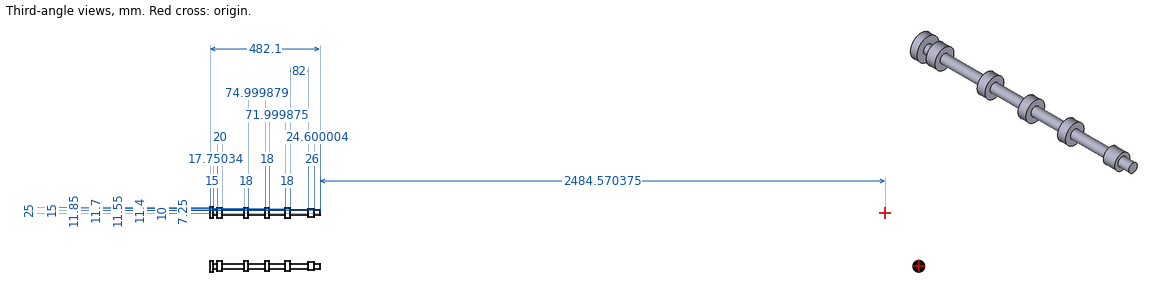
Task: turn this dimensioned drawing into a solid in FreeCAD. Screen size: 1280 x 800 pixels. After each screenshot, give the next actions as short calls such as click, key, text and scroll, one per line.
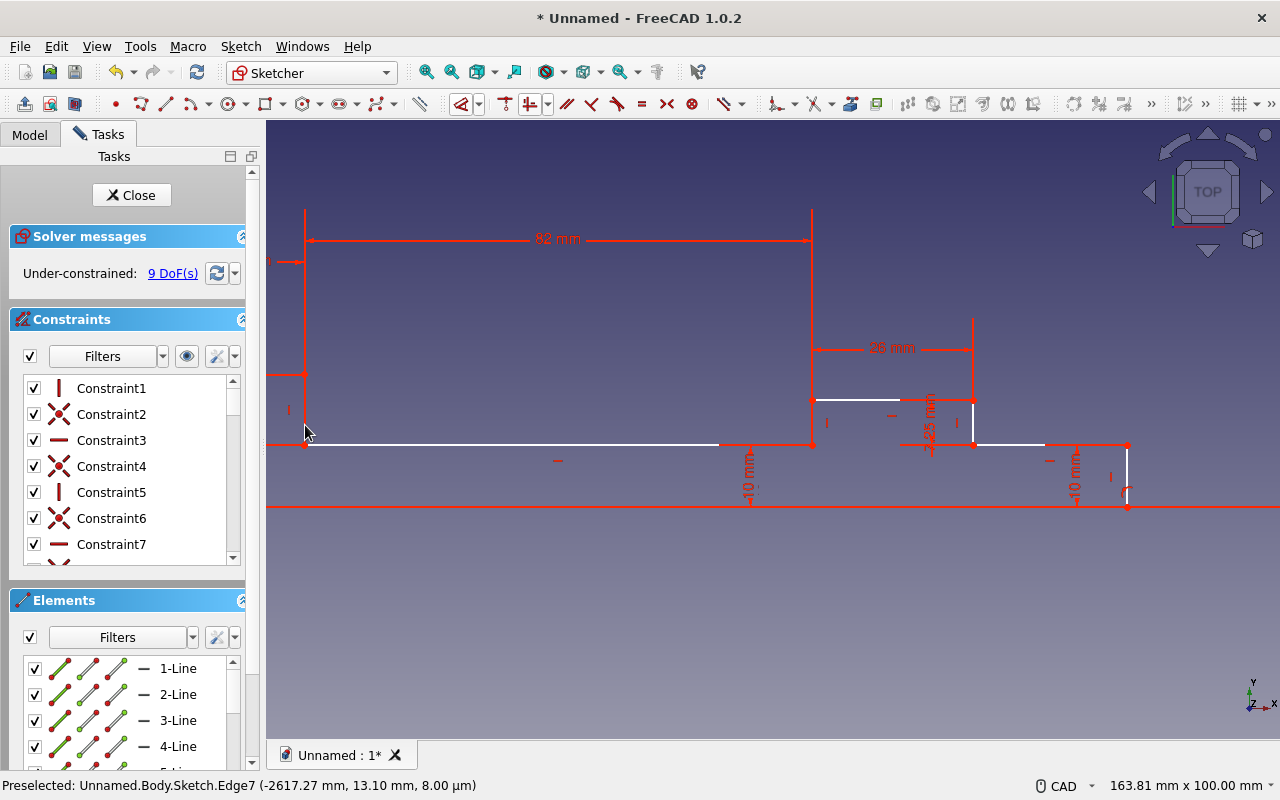
scroll(975, 429, down, 8)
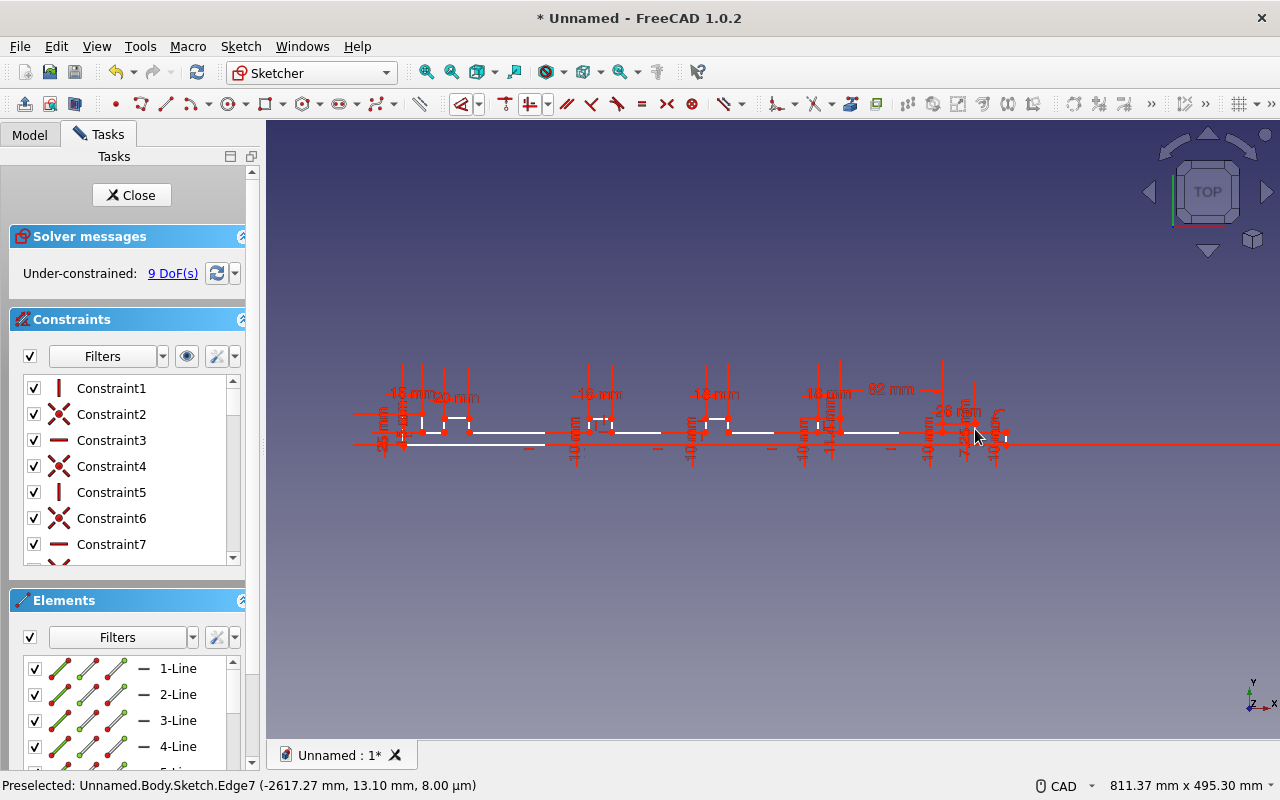
scroll(612, 429, up, 7)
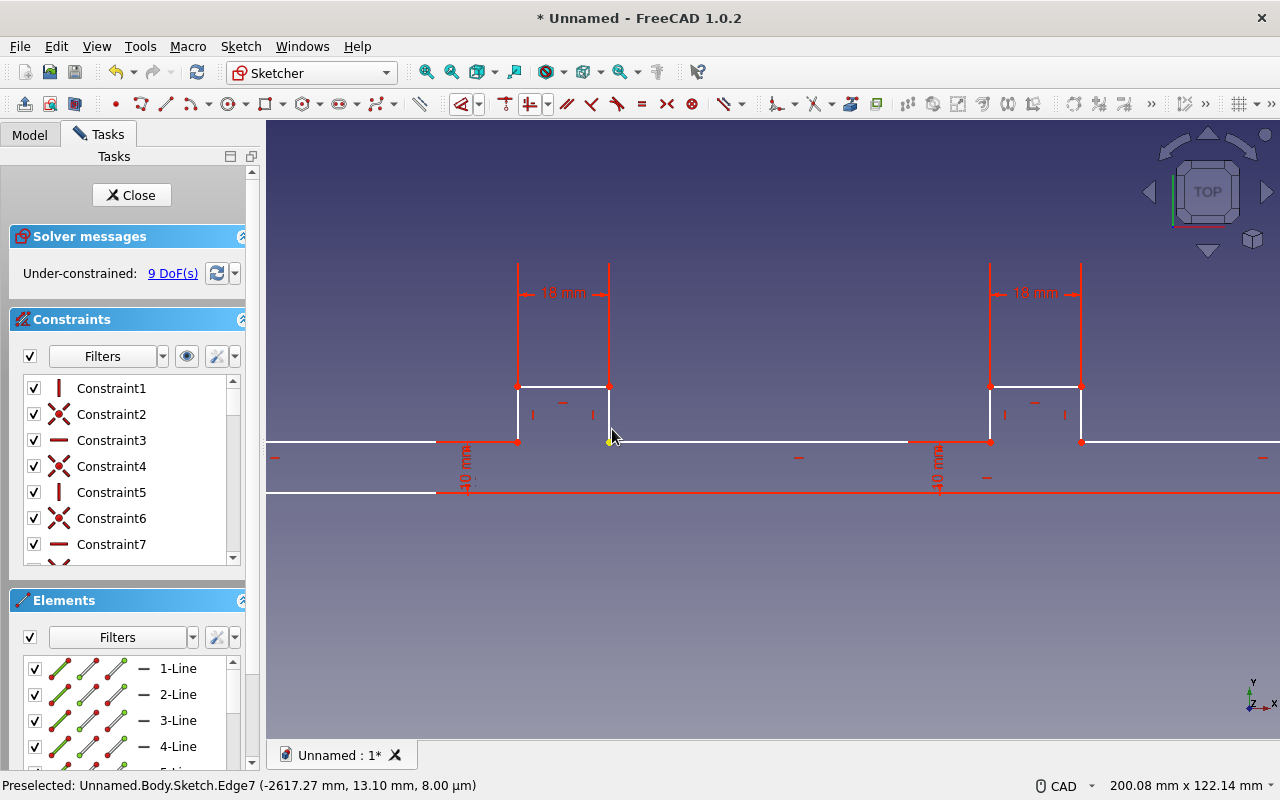
click(609, 426)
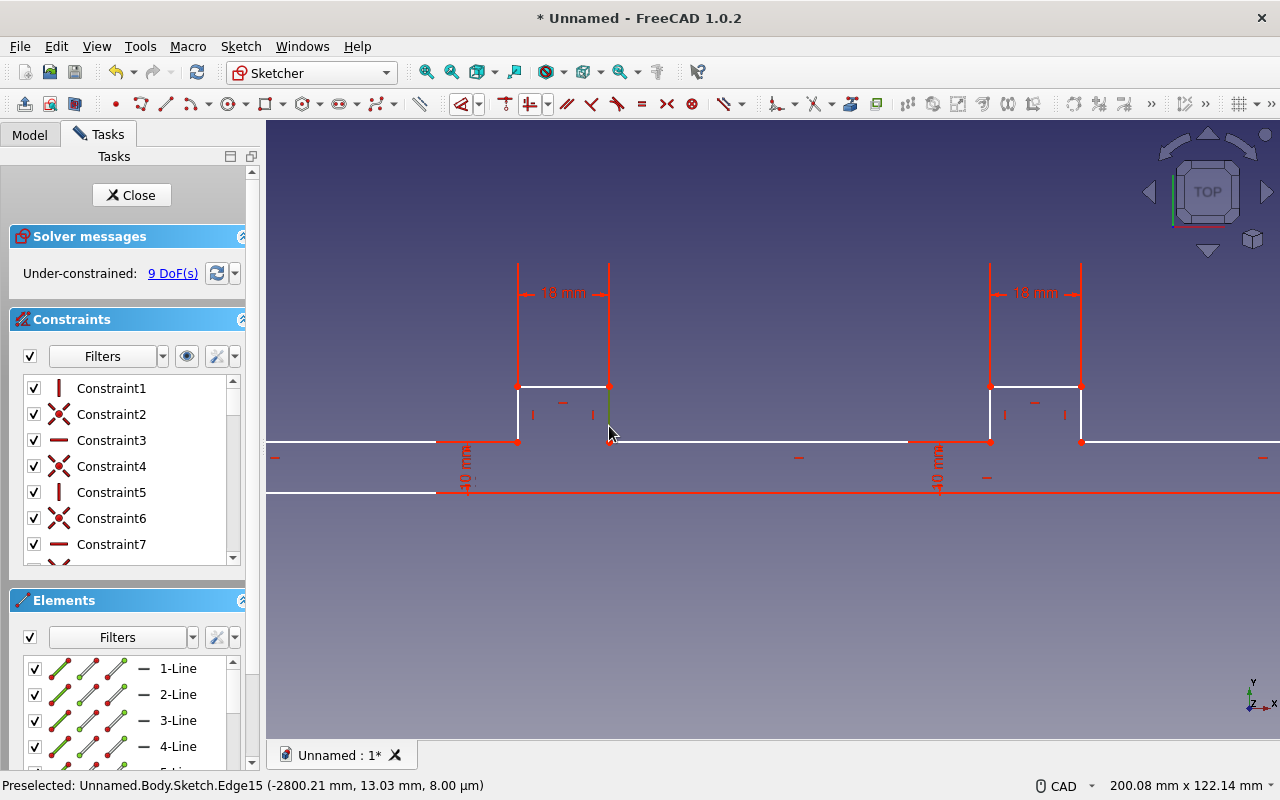
key(i)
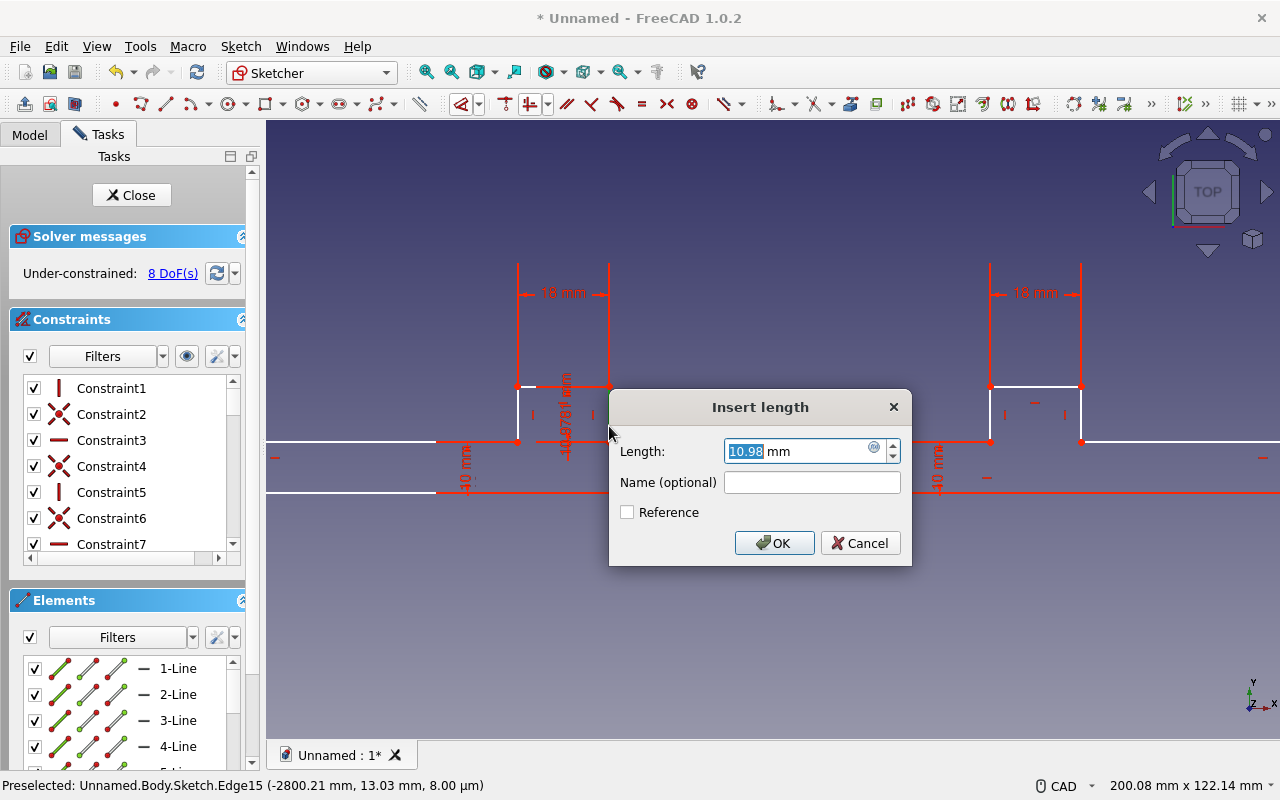
text(11.7)
key(Return)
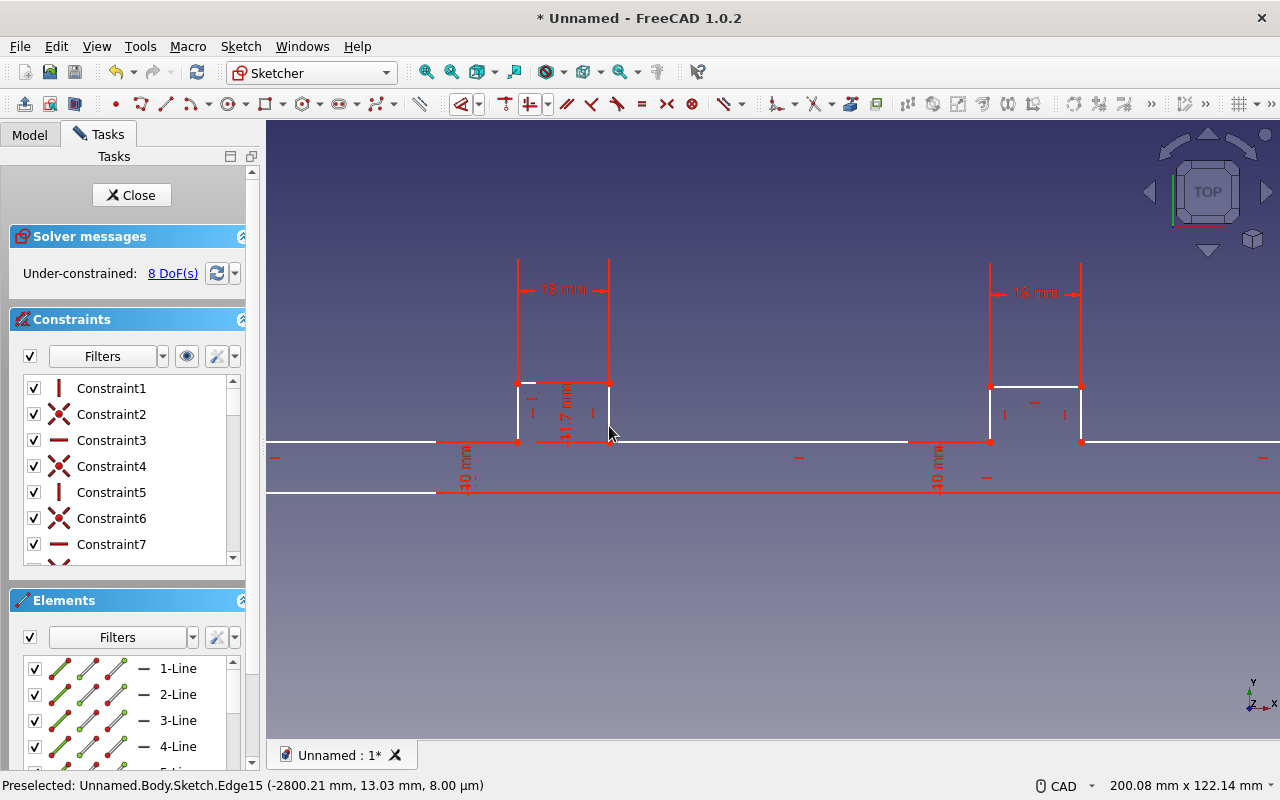
click(1081, 426)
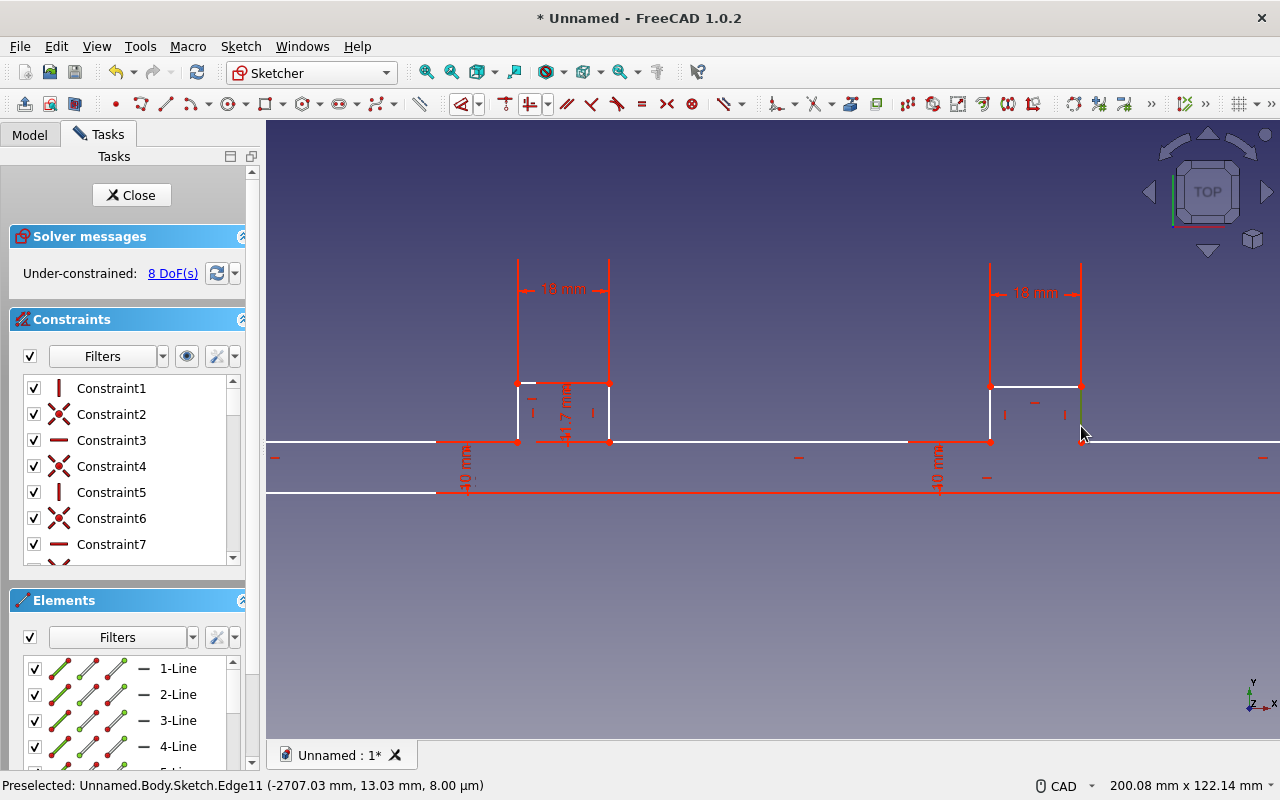
click(478, 104)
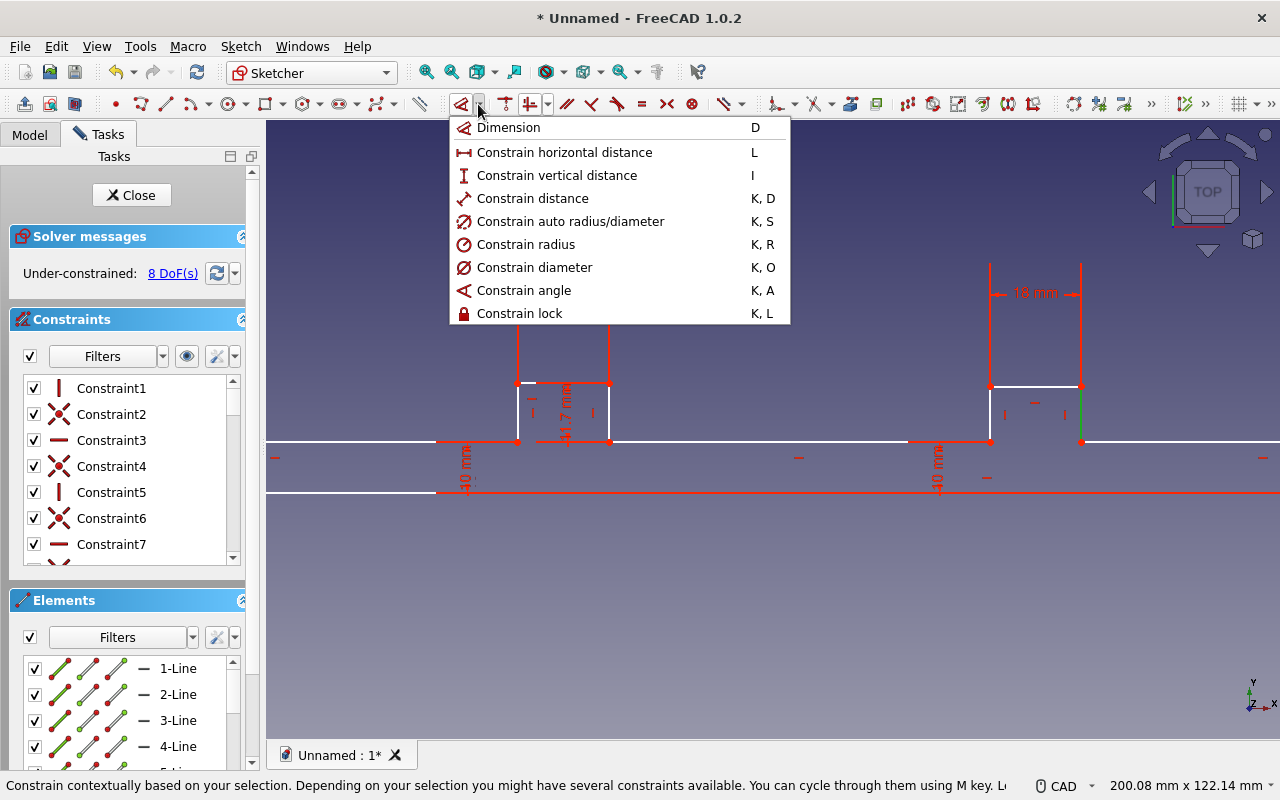
click(620, 176)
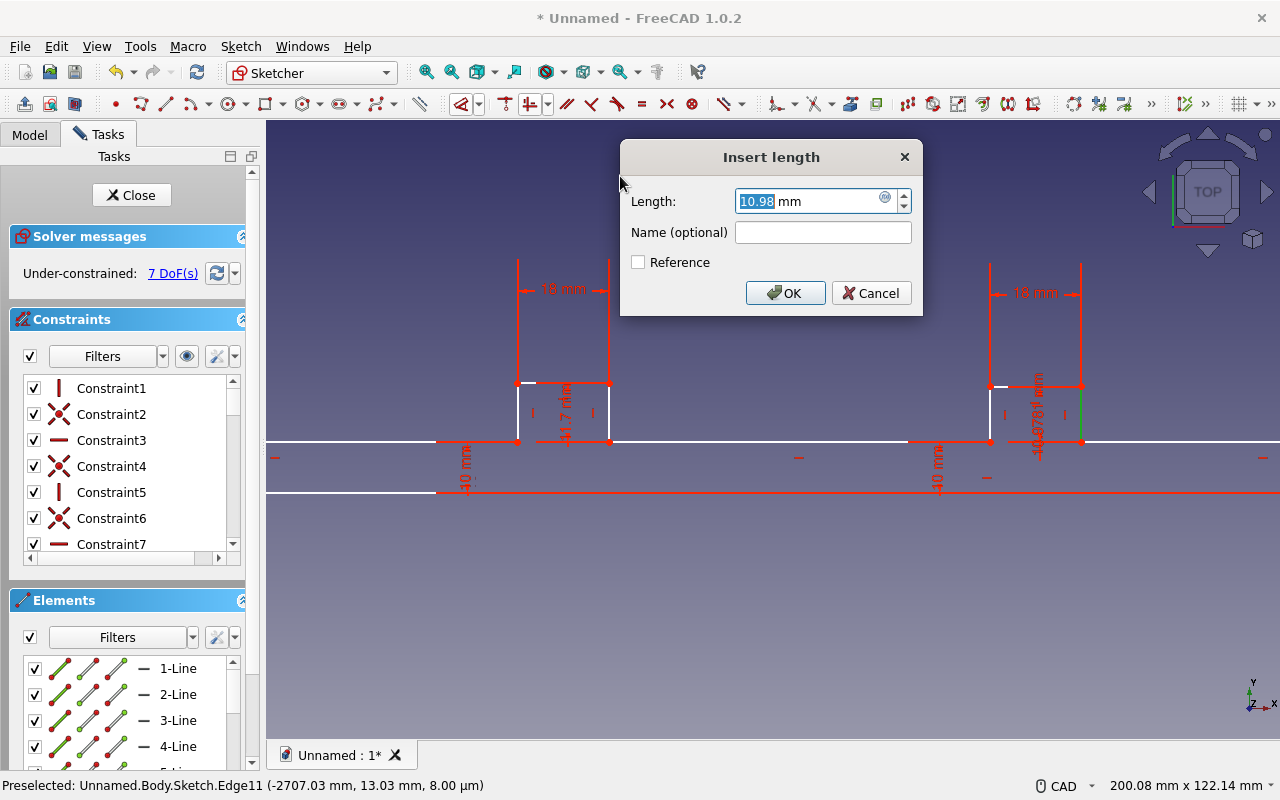
text(11.55)
key(Return)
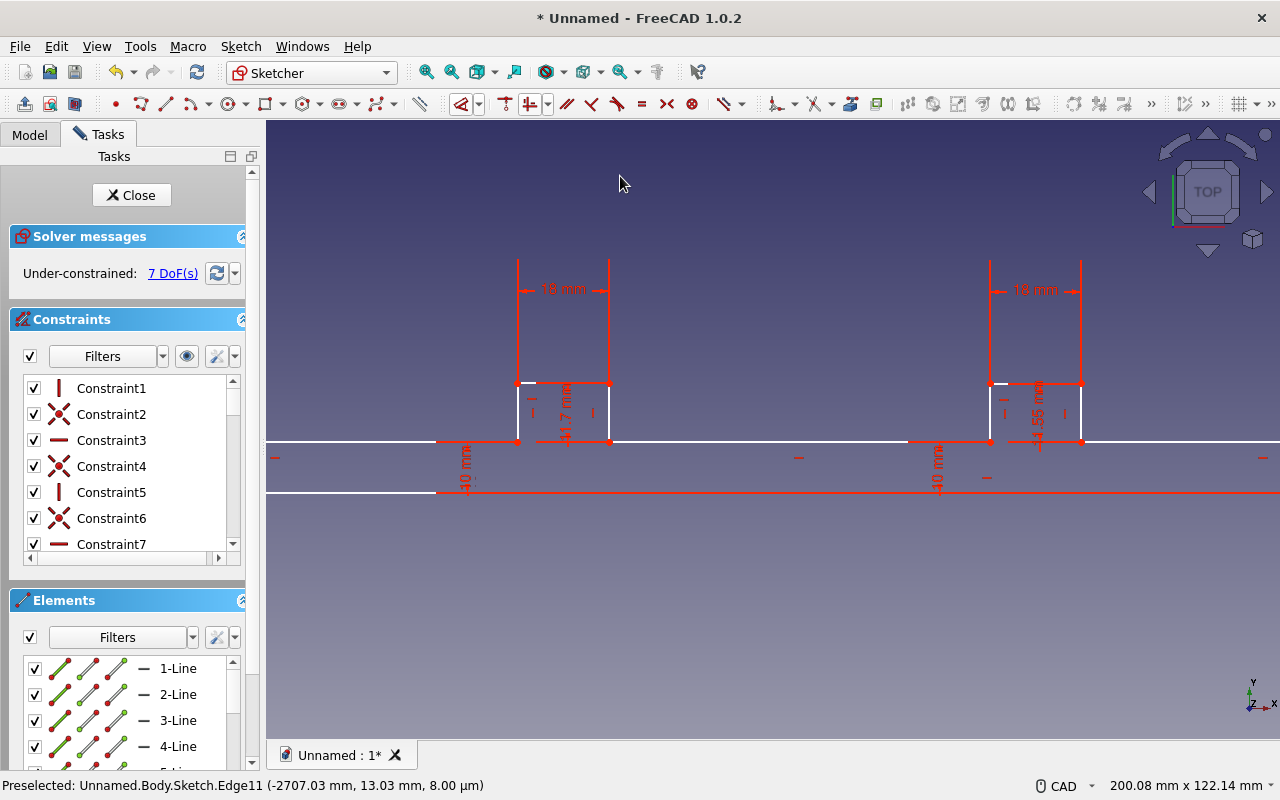
scroll(612, 429, down, 7)